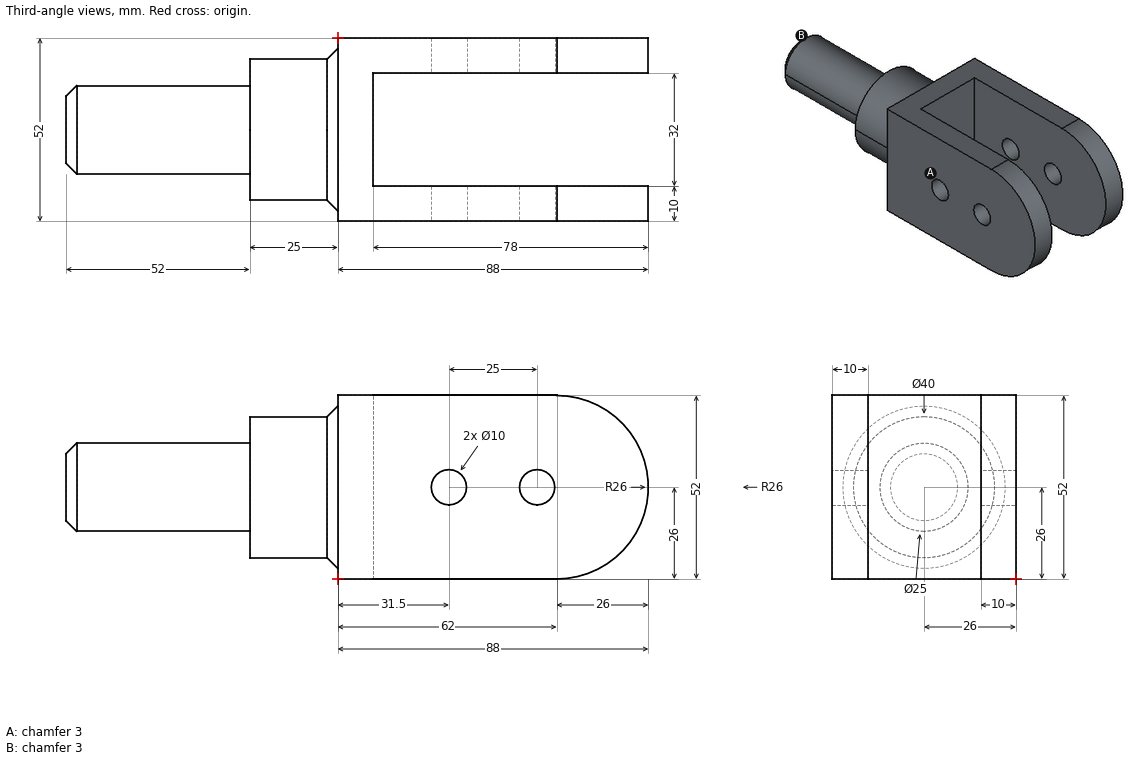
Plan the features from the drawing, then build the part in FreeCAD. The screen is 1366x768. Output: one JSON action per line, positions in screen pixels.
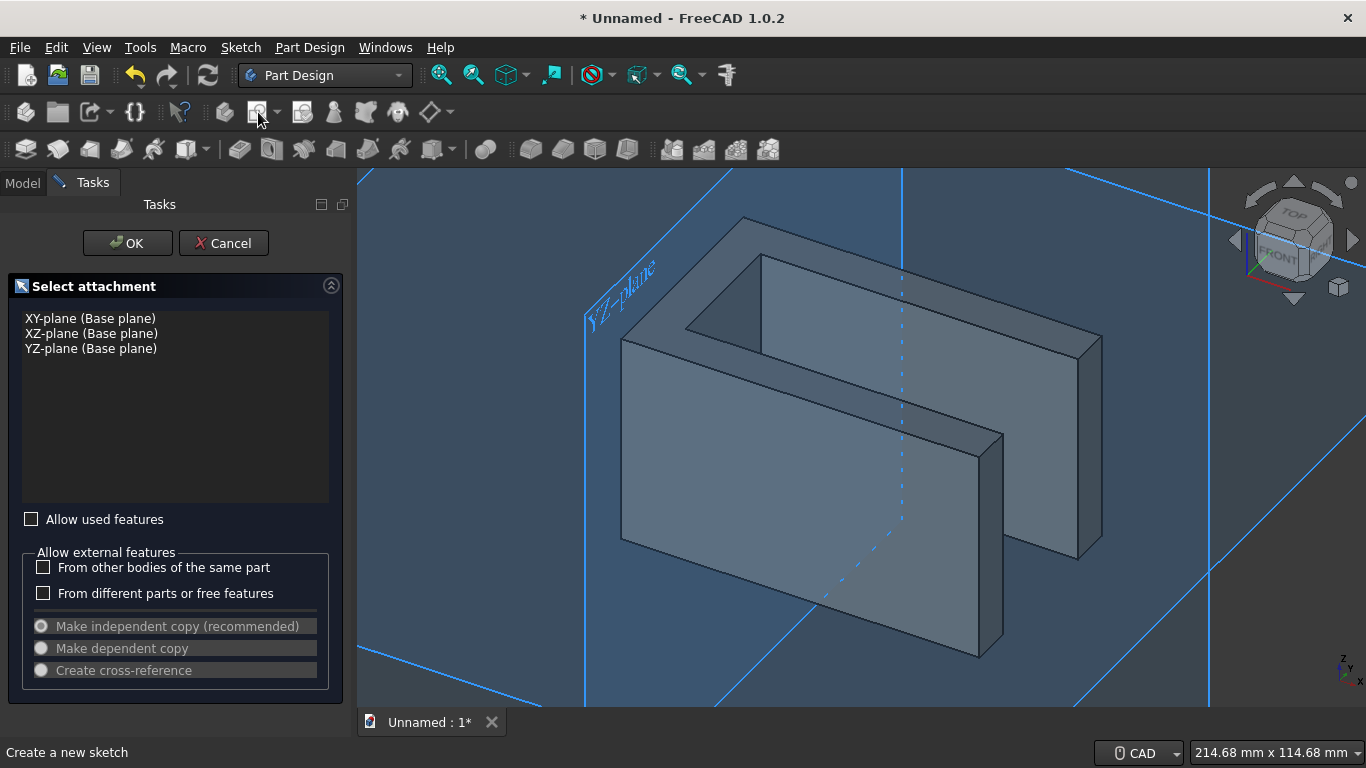
{"action": "left_click", "coordinate": [82, 334]}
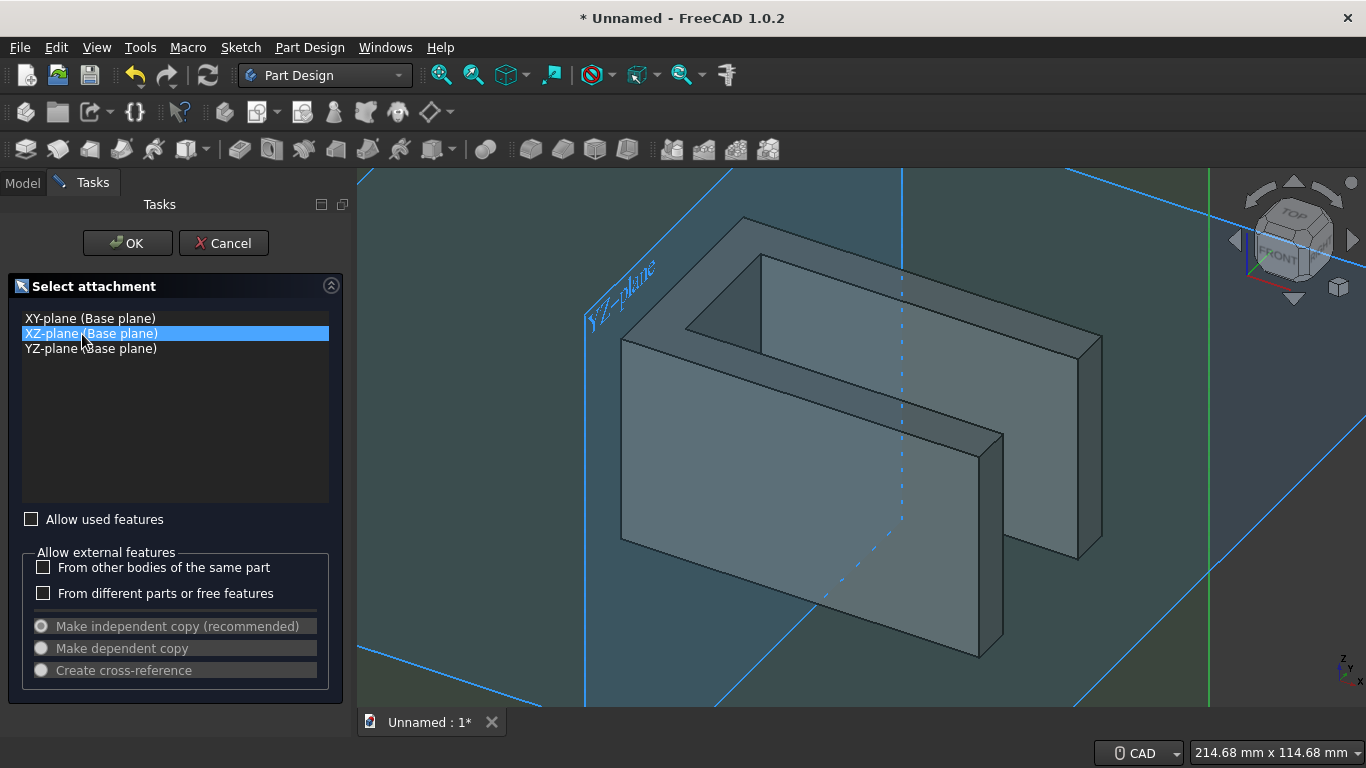
{"action": "left_click", "coordinate": [128, 243]}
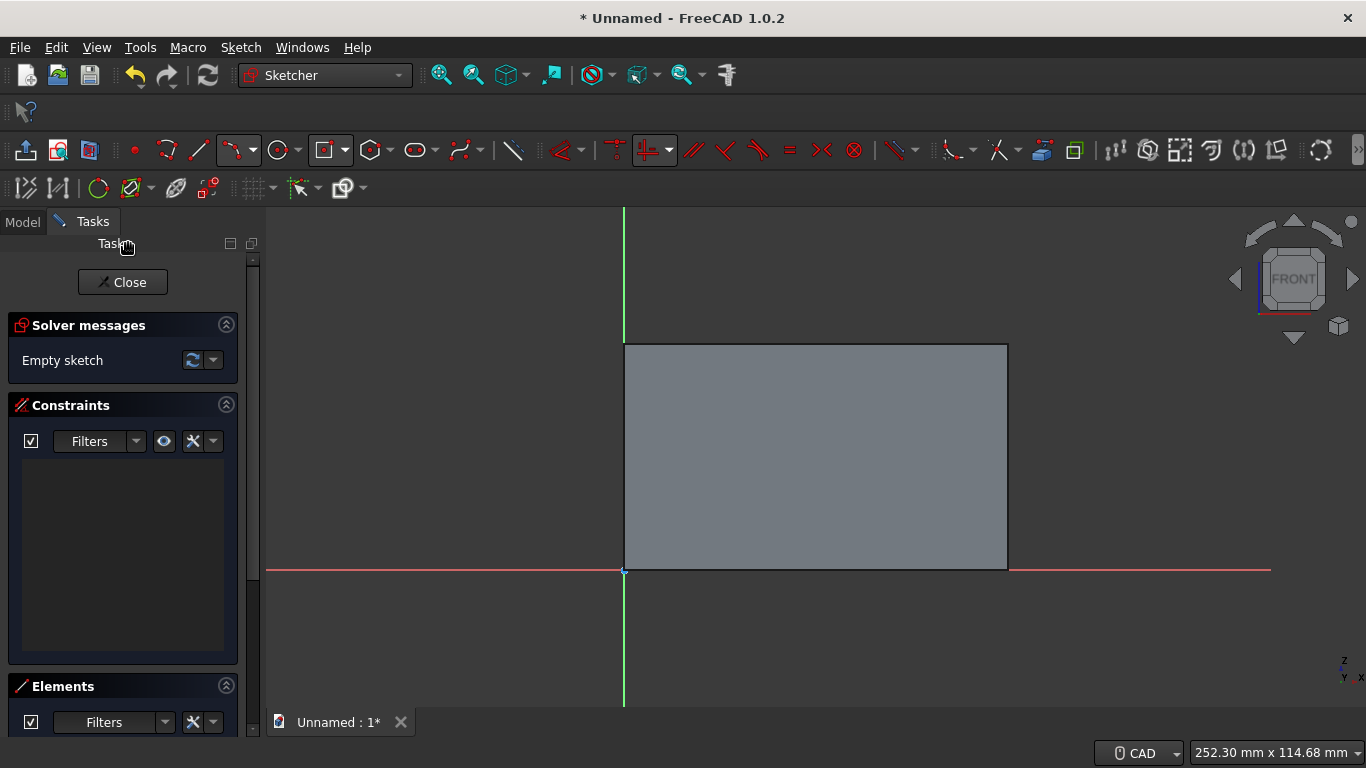
{"action": "left_click", "coordinate": [90, 150]}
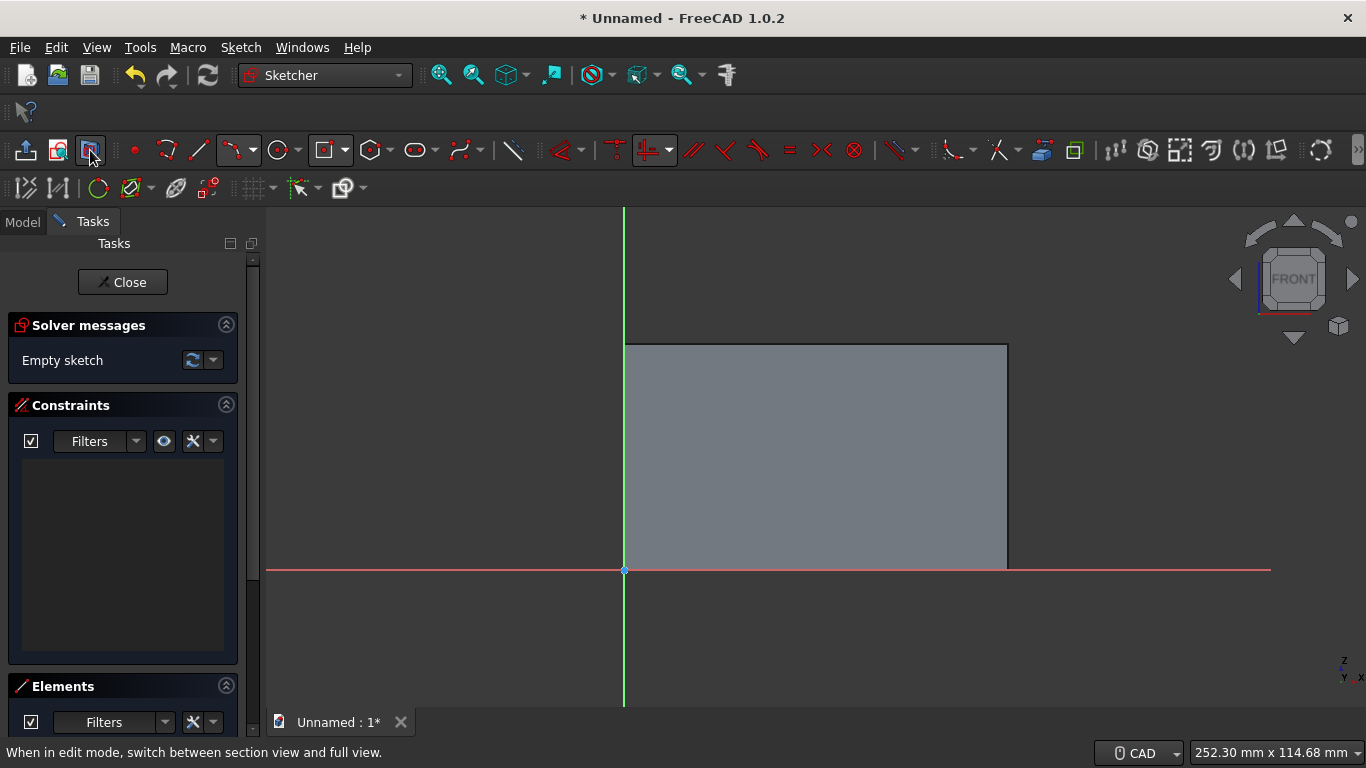
{"action": "left_click", "coordinate": [200, 150]}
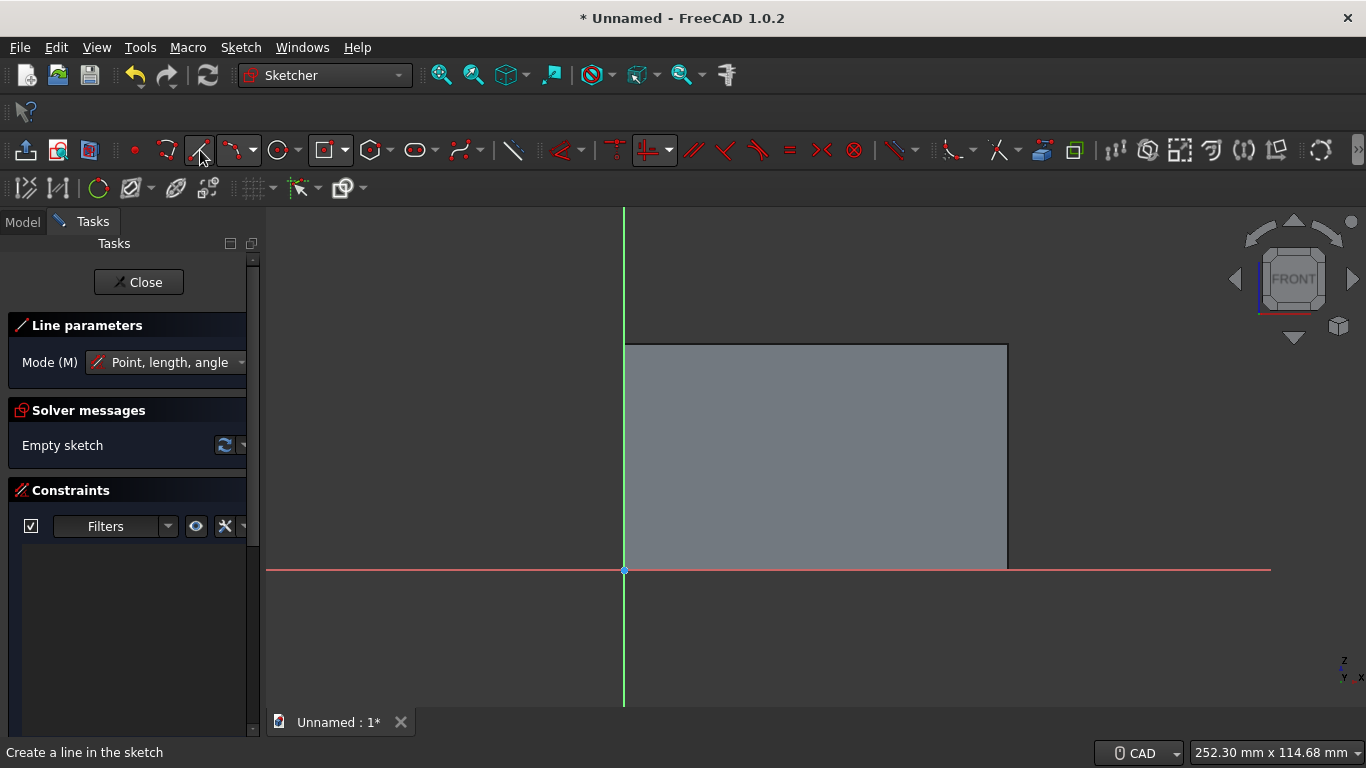
{"action": "left_click", "coordinate": [1008, 570]}
{"action": "left_click", "coordinate": [1008, 344]}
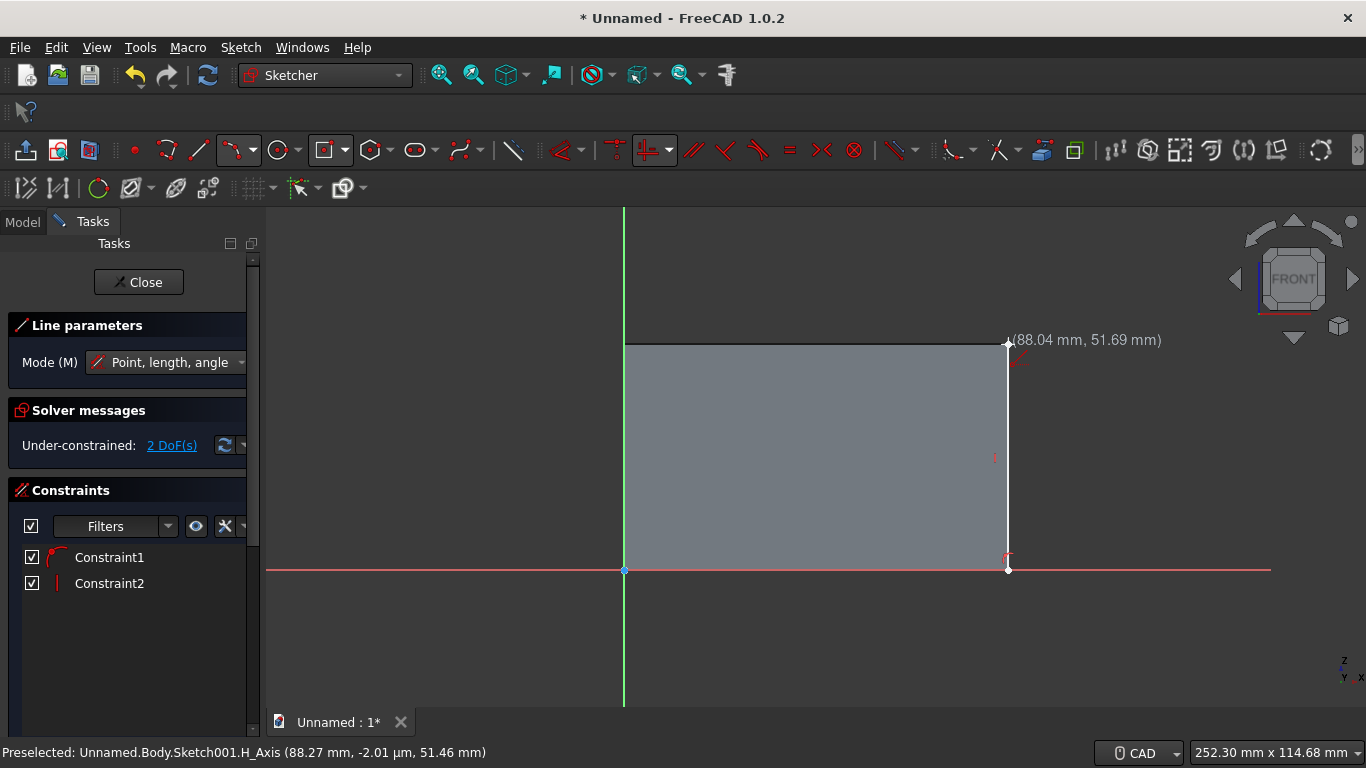
{"action": "left_click", "coordinate": [232, 150]}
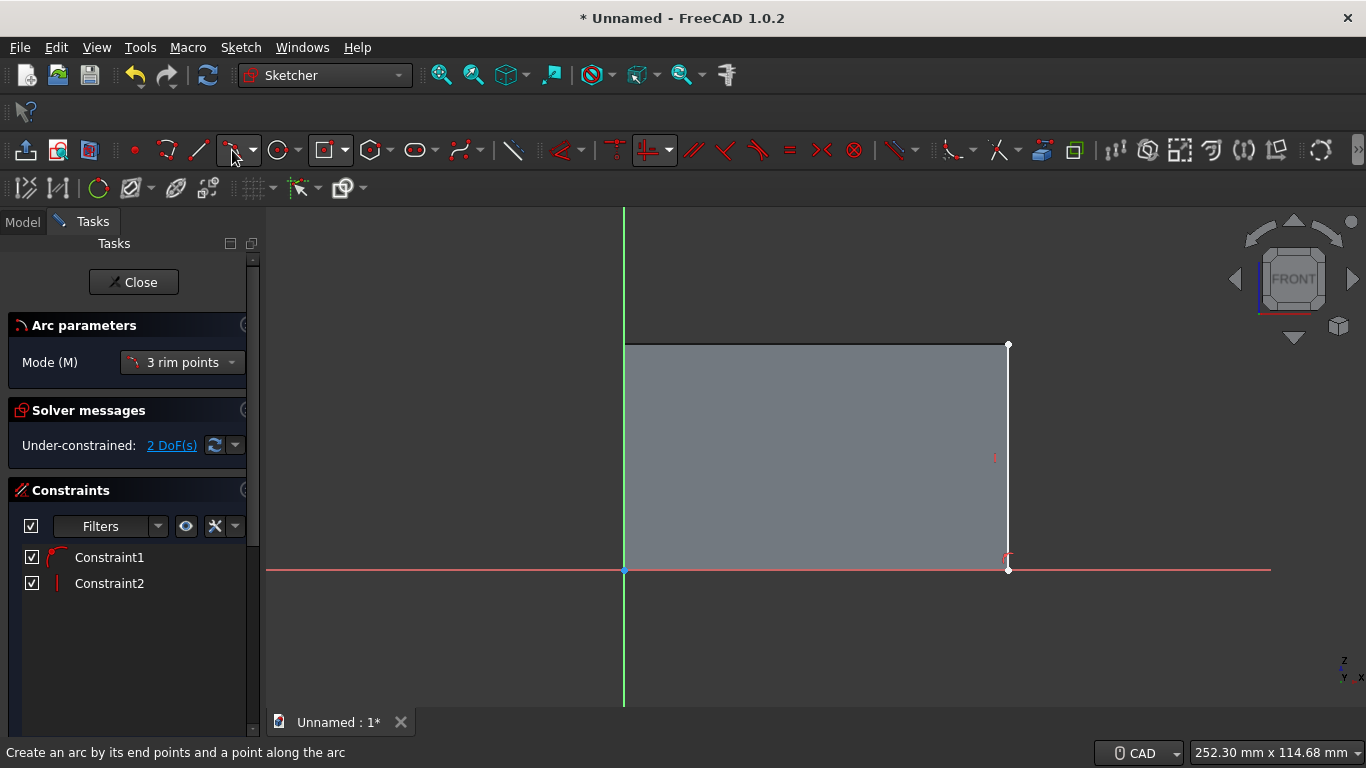
{"action": "left_click", "coordinate": [1008, 345]}
{"action": "left_click", "coordinate": [1008, 570]}
{"action": "left_click", "coordinate": [1121, 457]}
{"action": "key", "text": "Escape"}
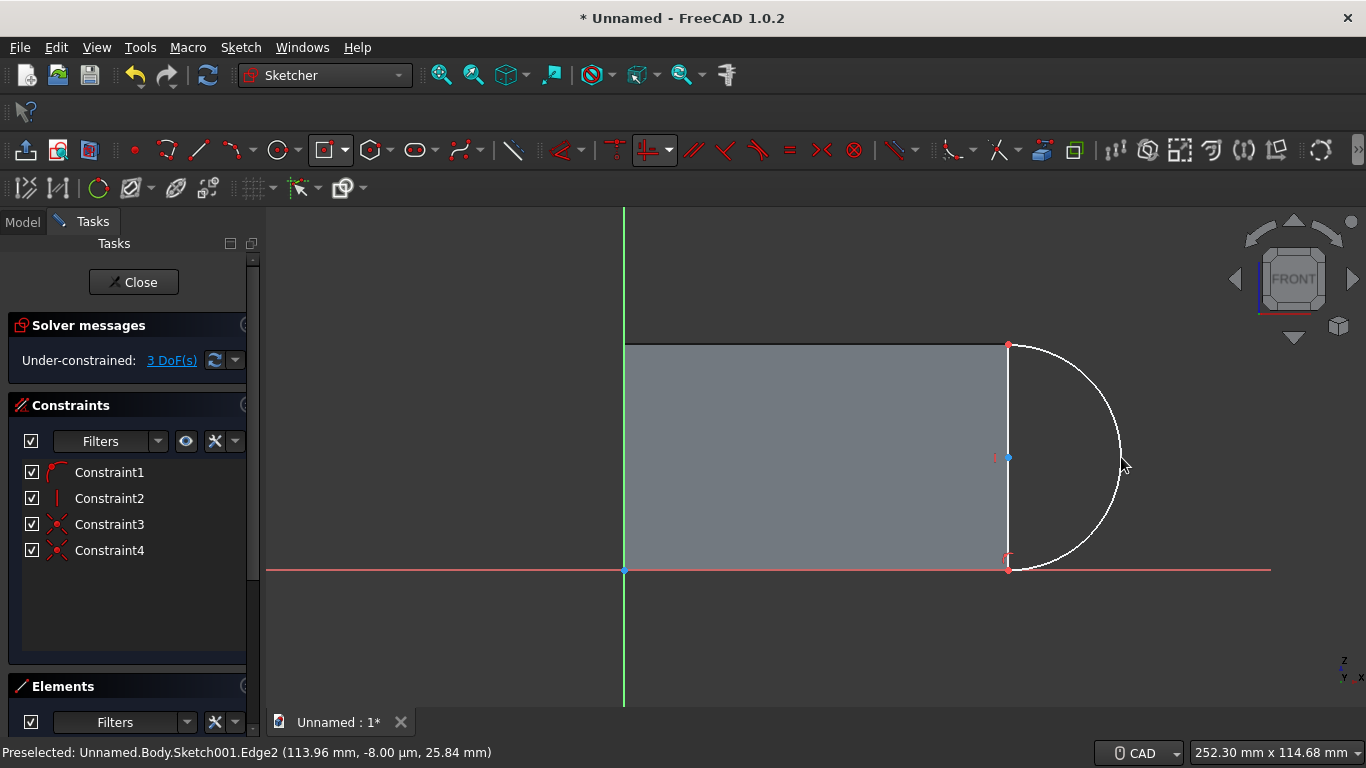
{"action": "left_click", "coordinate": [560, 150]}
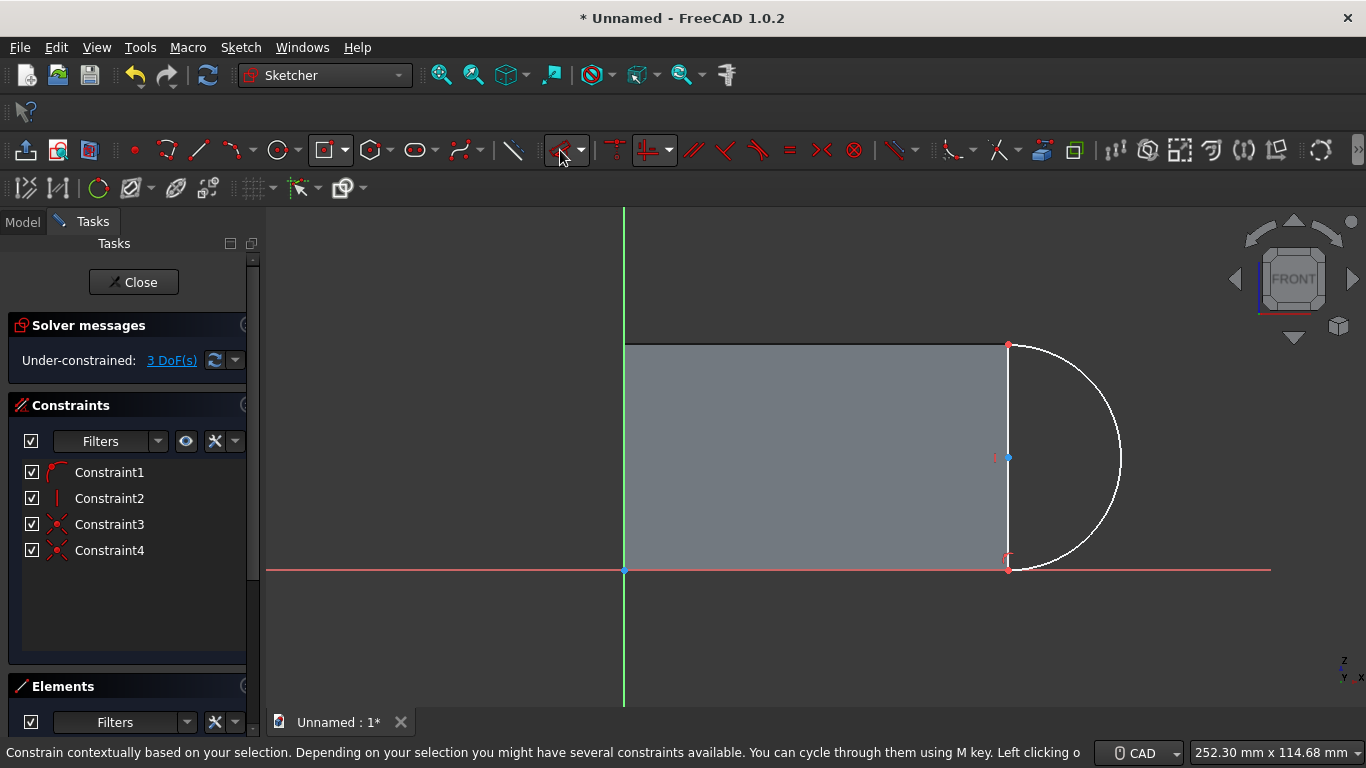
{"action": "left_click", "coordinate": [1099, 524]}
{"action": "left_click", "coordinate": [1125, 543]}